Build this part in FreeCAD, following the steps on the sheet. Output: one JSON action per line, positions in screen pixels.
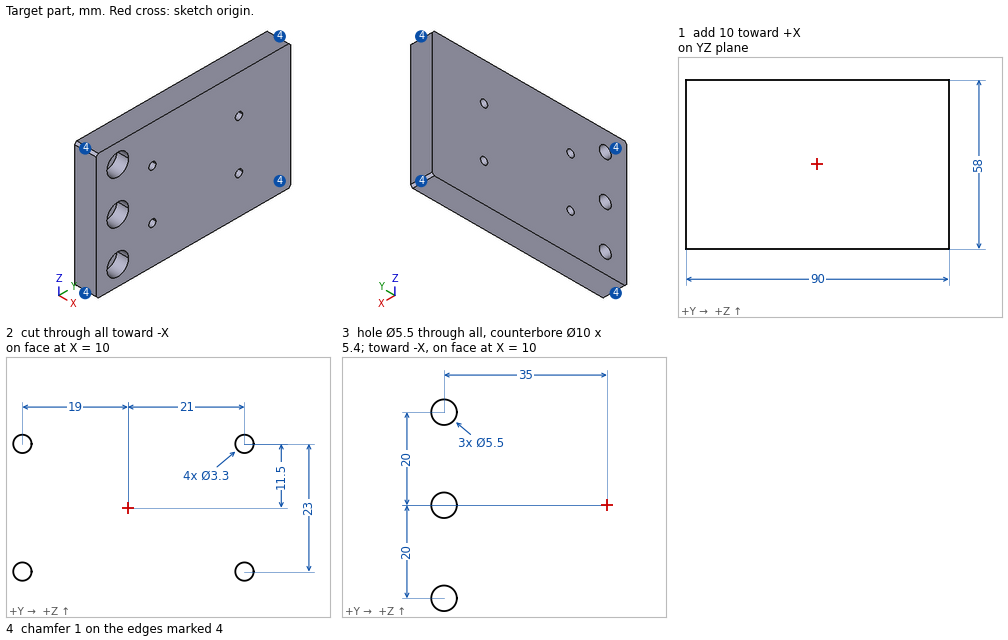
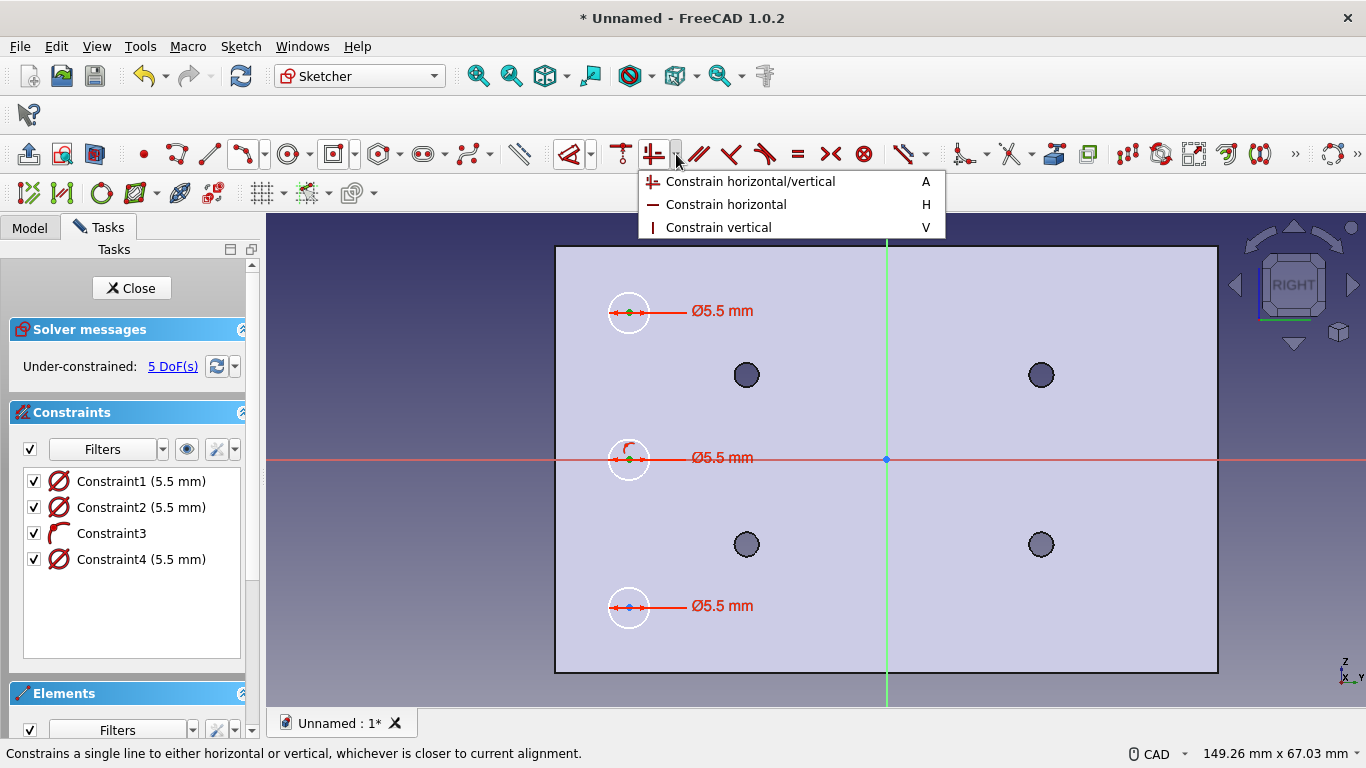
{"action": "left_click", "coordinate": [792, 228]}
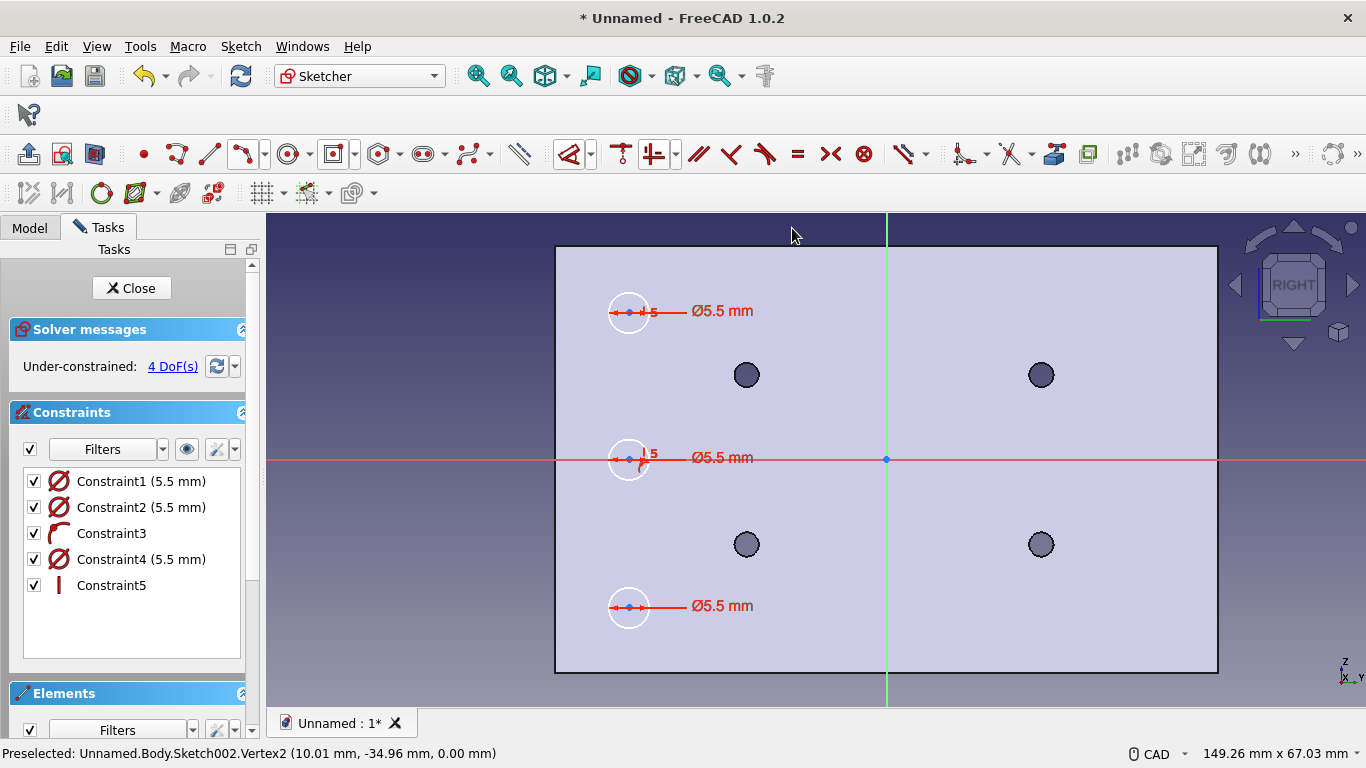
{"action": "left_click", "coordinate": [629, 460]}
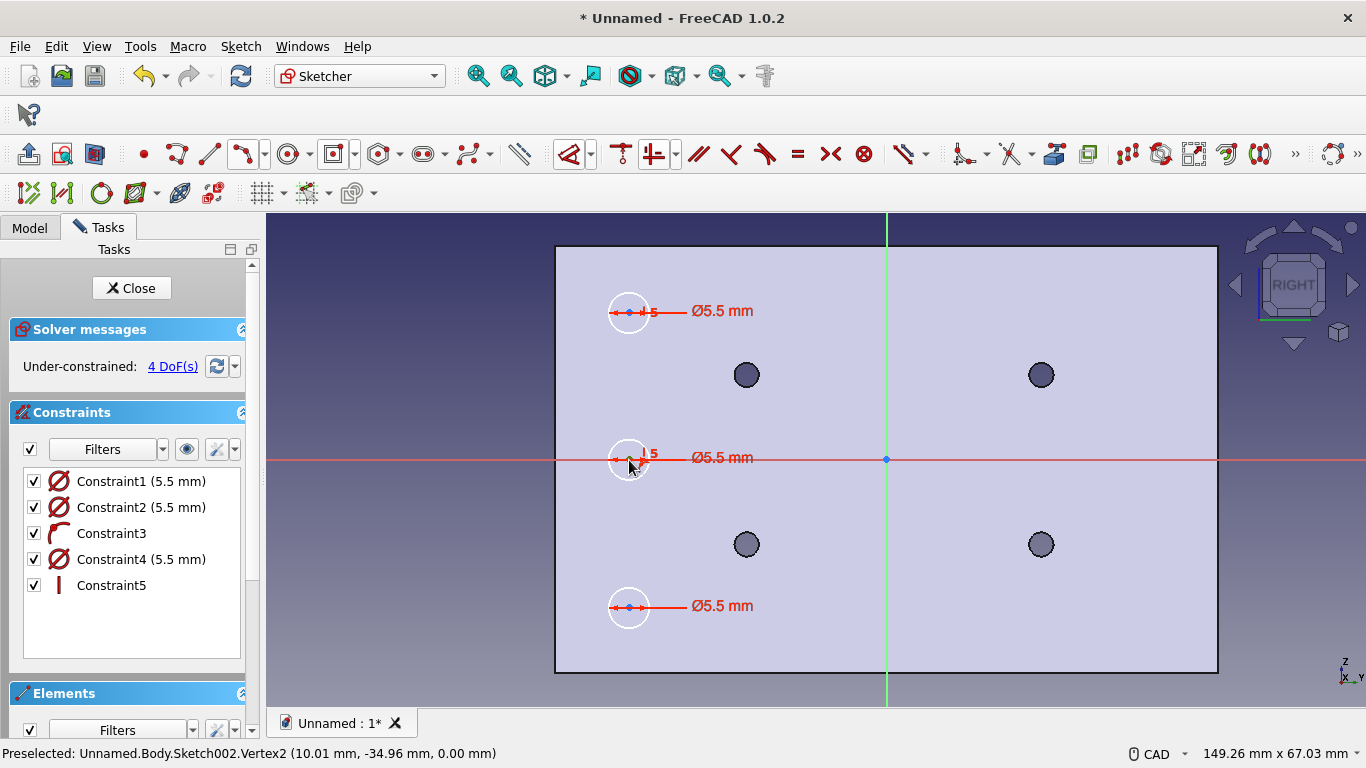
{"action": "left_click", "coordinate": [629, 608]}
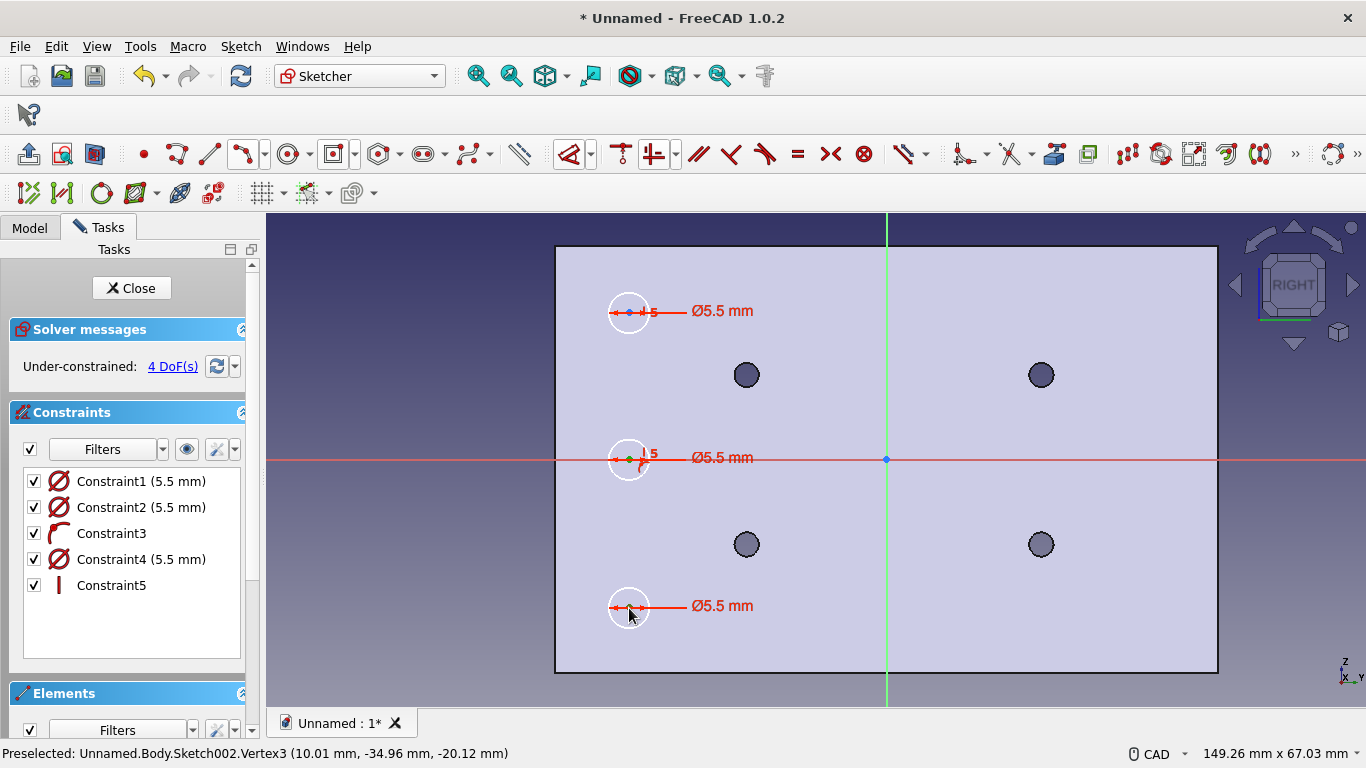
{"action": "left_click", "coordinate": [676, 154]}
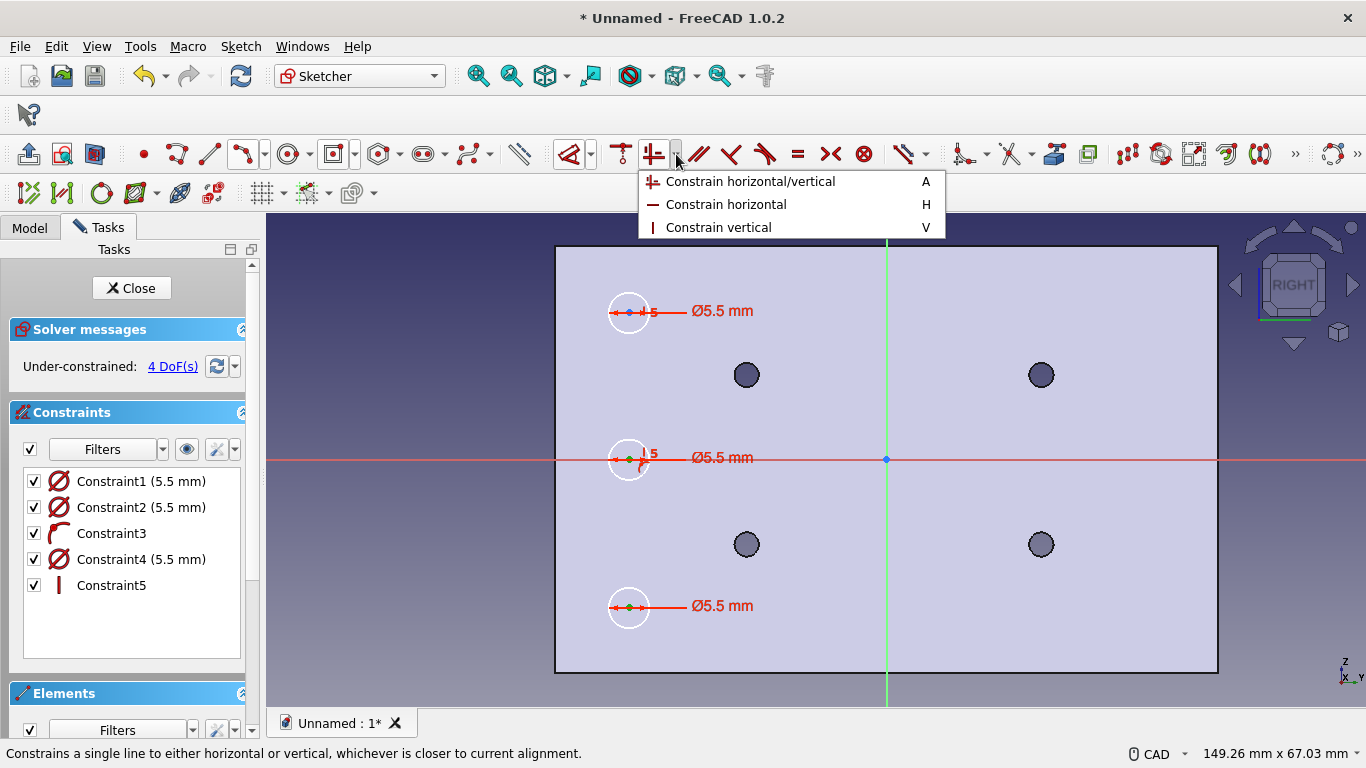
{"action": "left_click", "coordinate": [792, 228]}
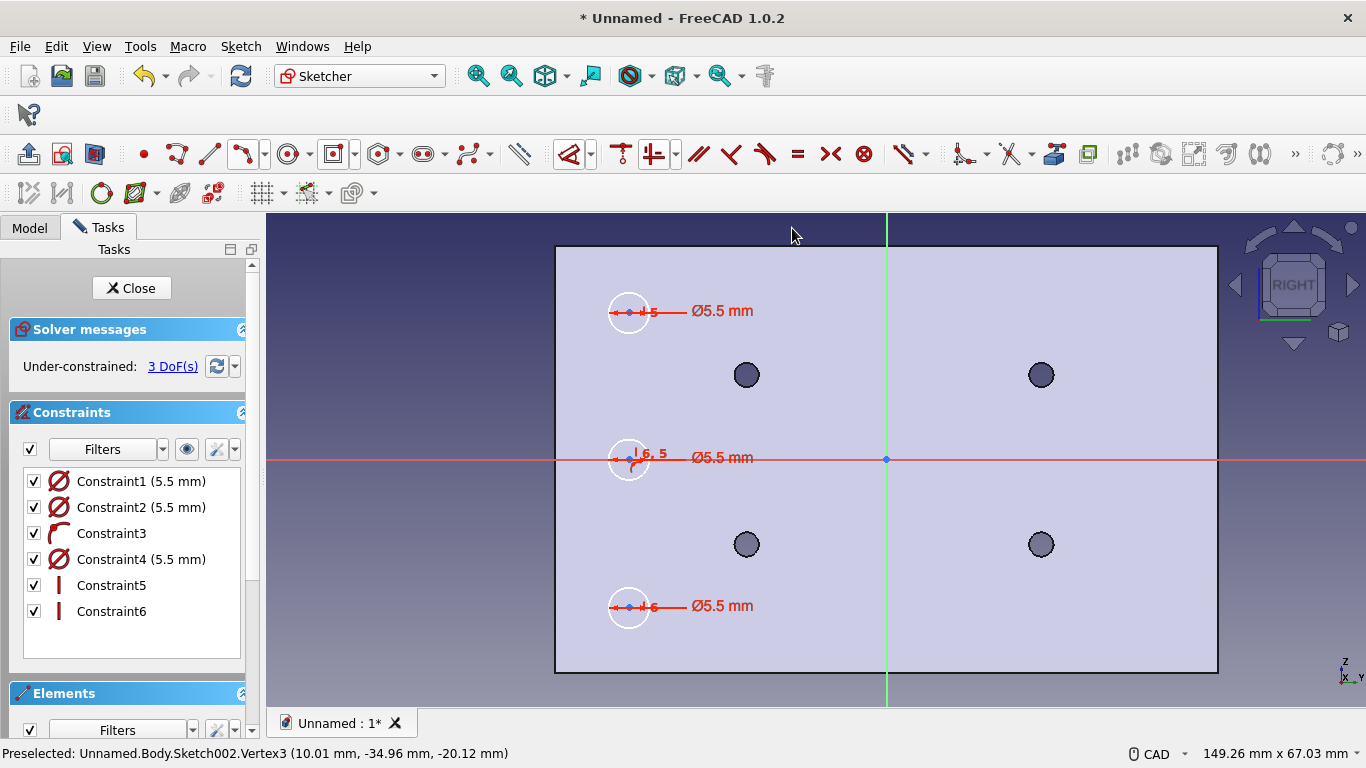
{"action": "left_click", "coordinate": [629, 313]}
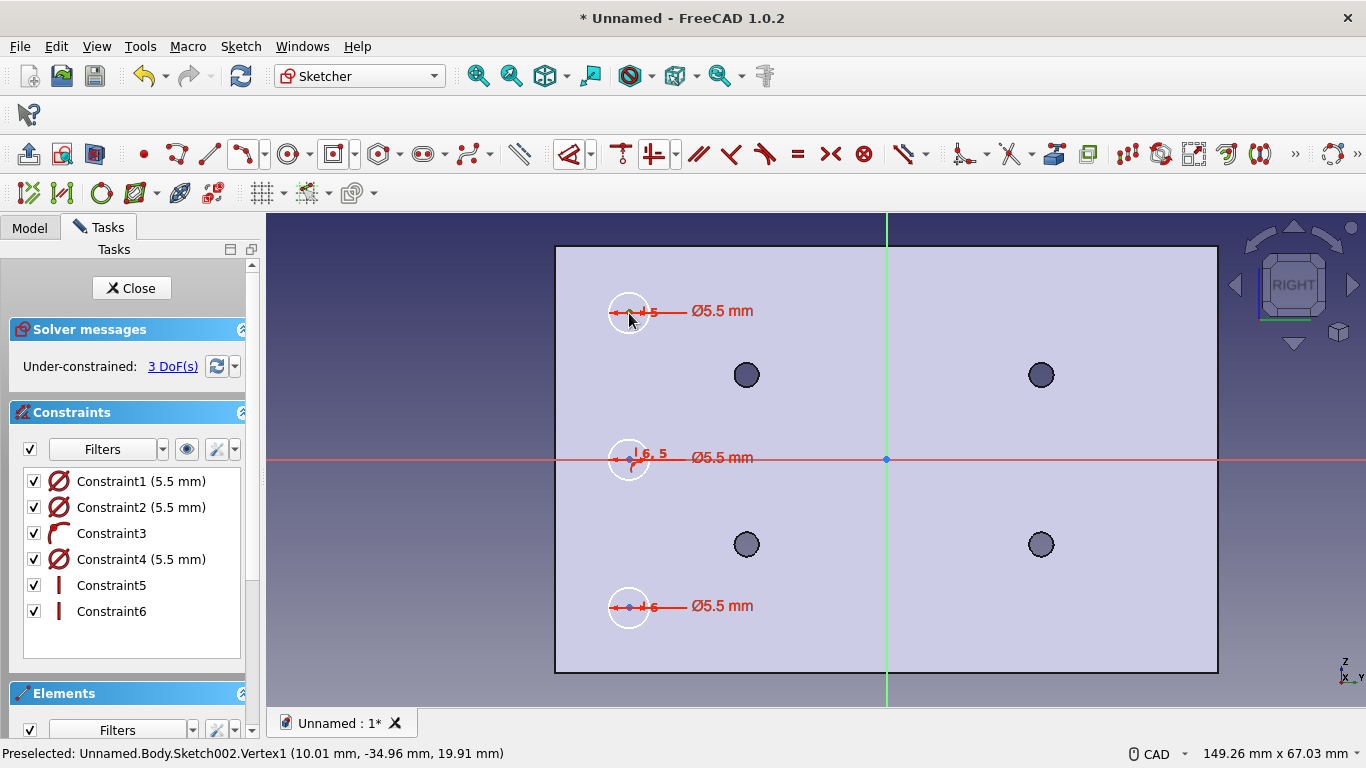
{"action": "left_click", "coordinate": [590, 154]}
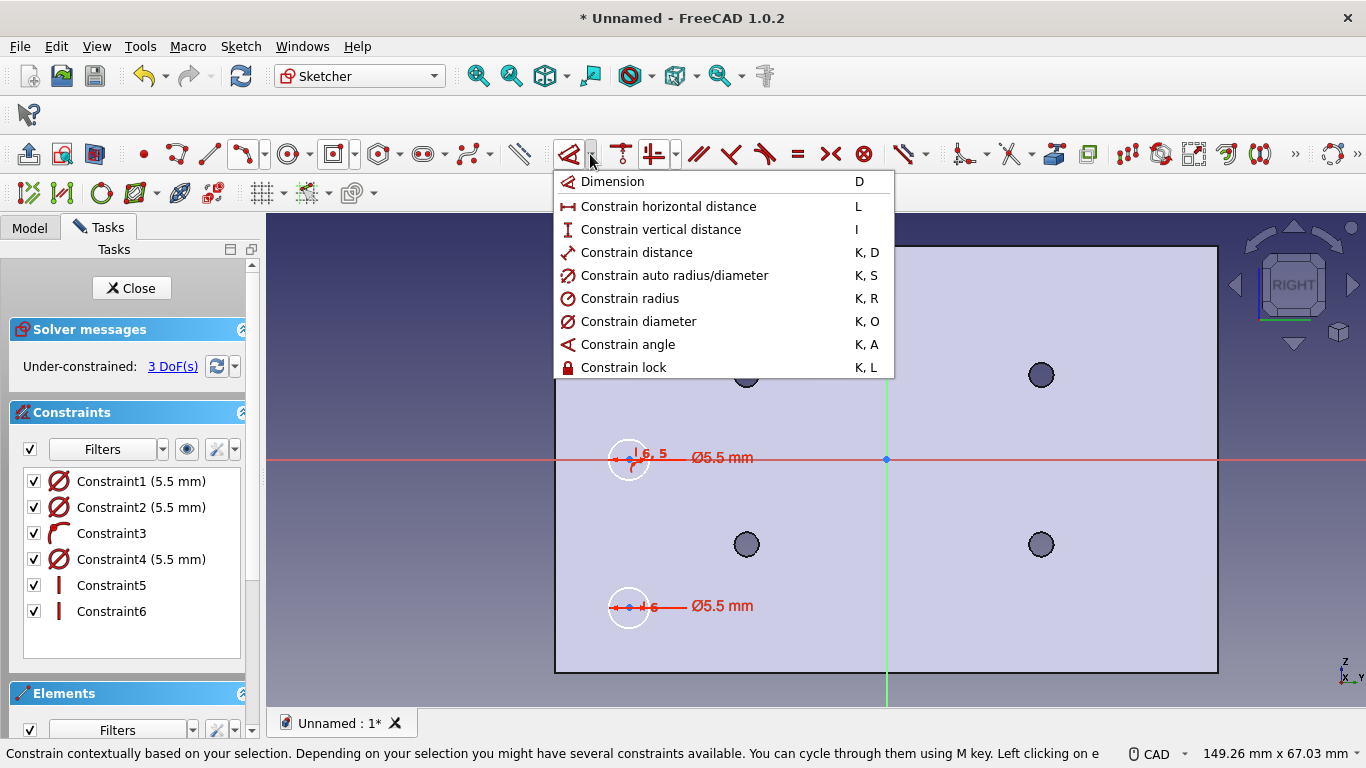
{"action": "left_click", "coordinate": [724, 206]}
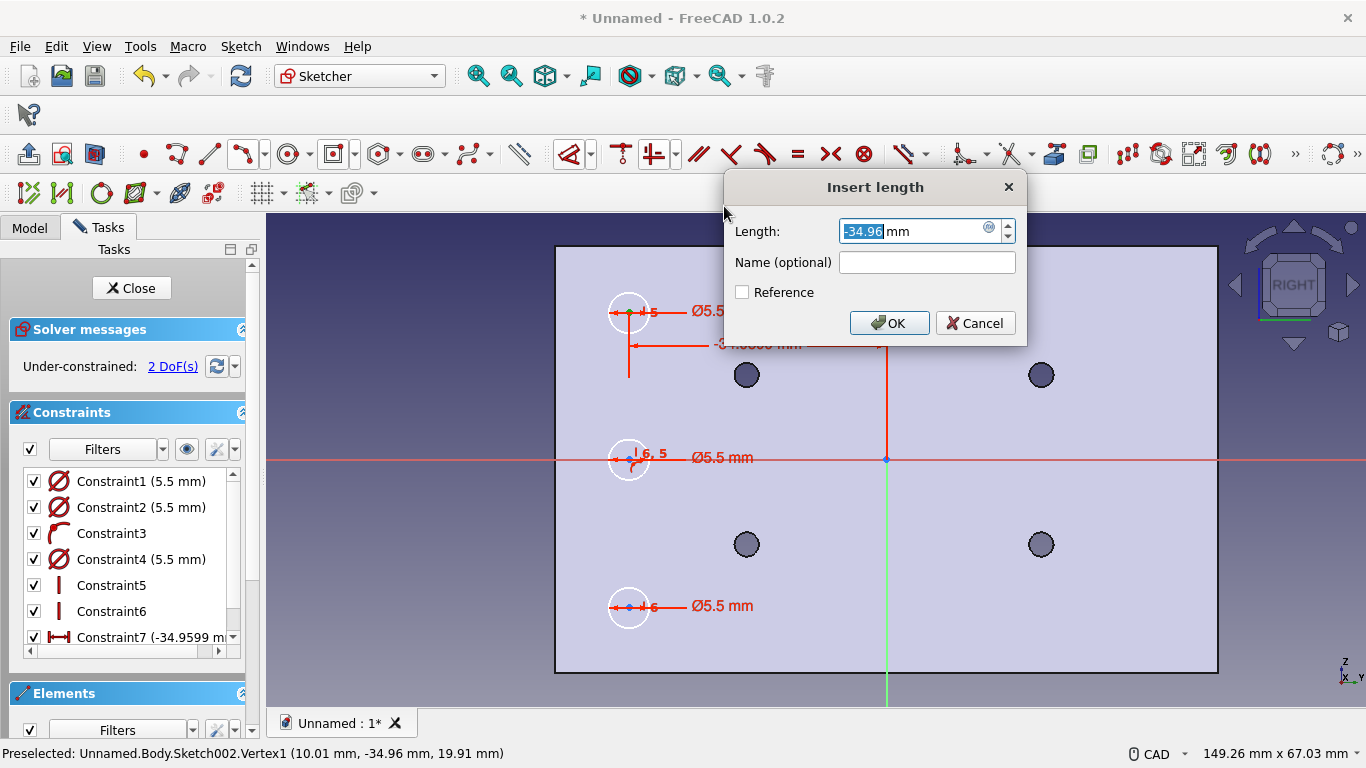
{"action": "type", "text": "-35"}
{"action": "key", "text": "Return"}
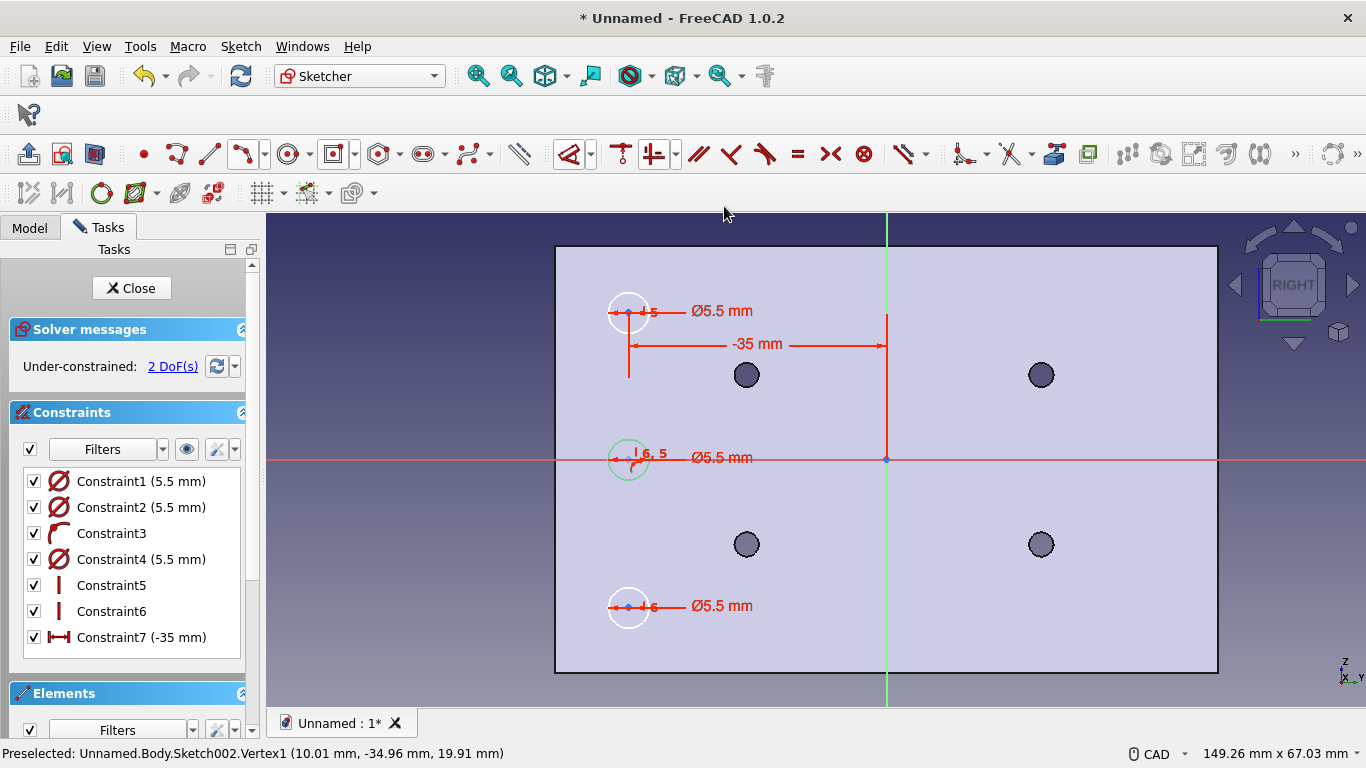
{"action": "left_click", "coordinate": [629, 313]}